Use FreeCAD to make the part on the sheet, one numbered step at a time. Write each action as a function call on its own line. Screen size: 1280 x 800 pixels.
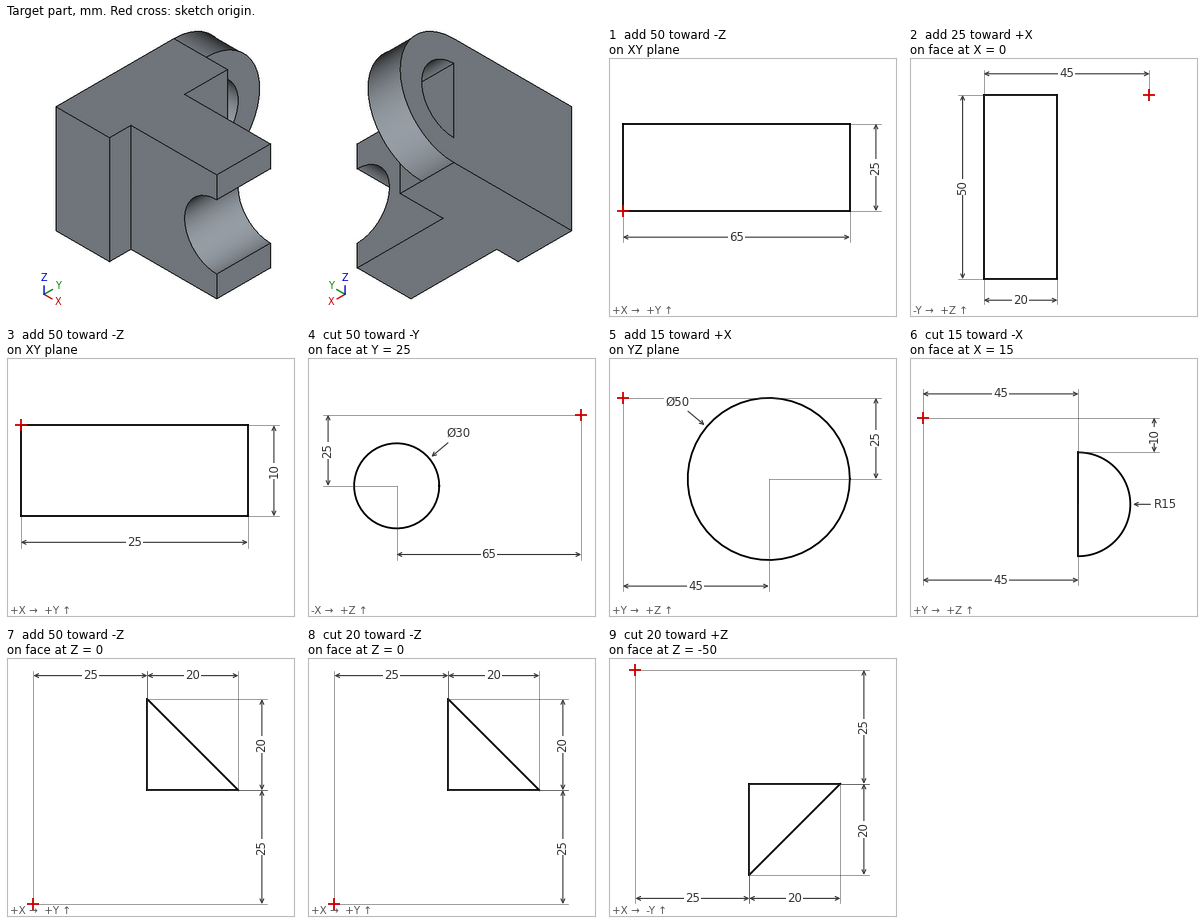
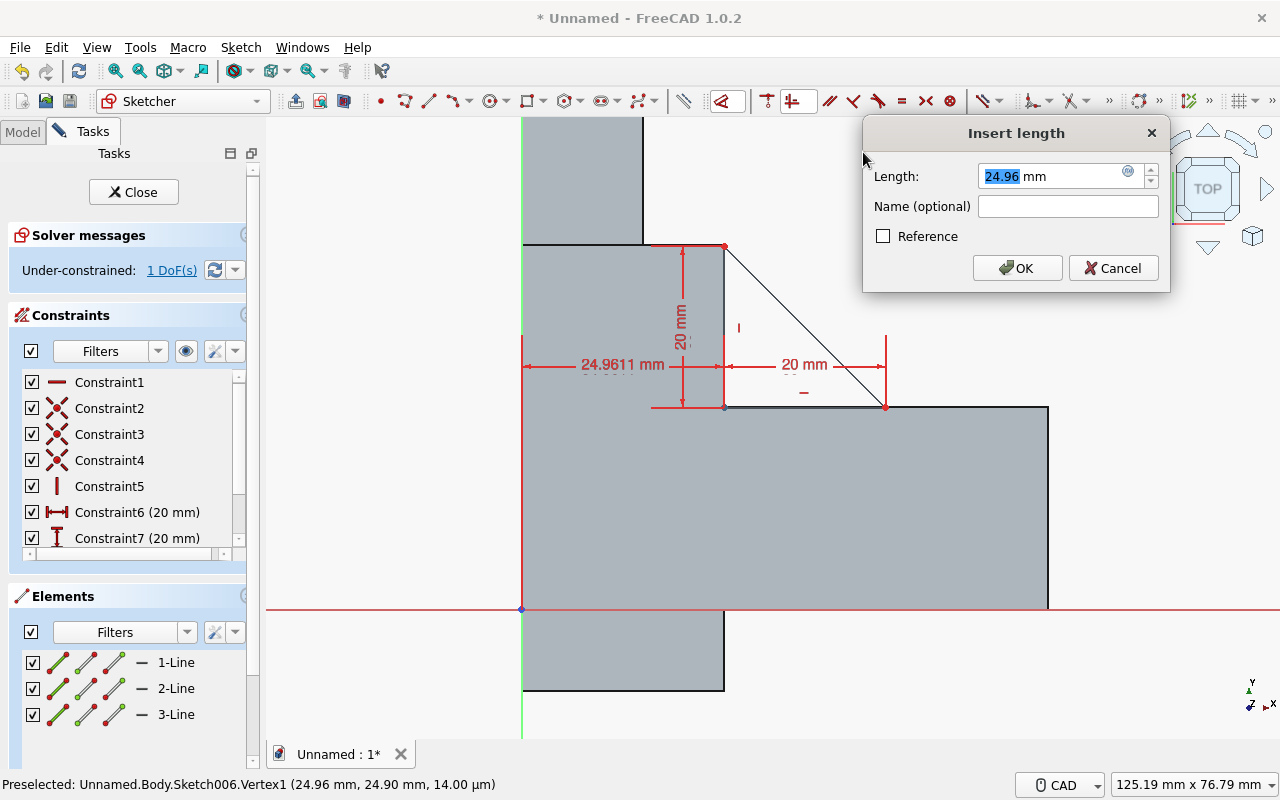
text(25)
key(Return)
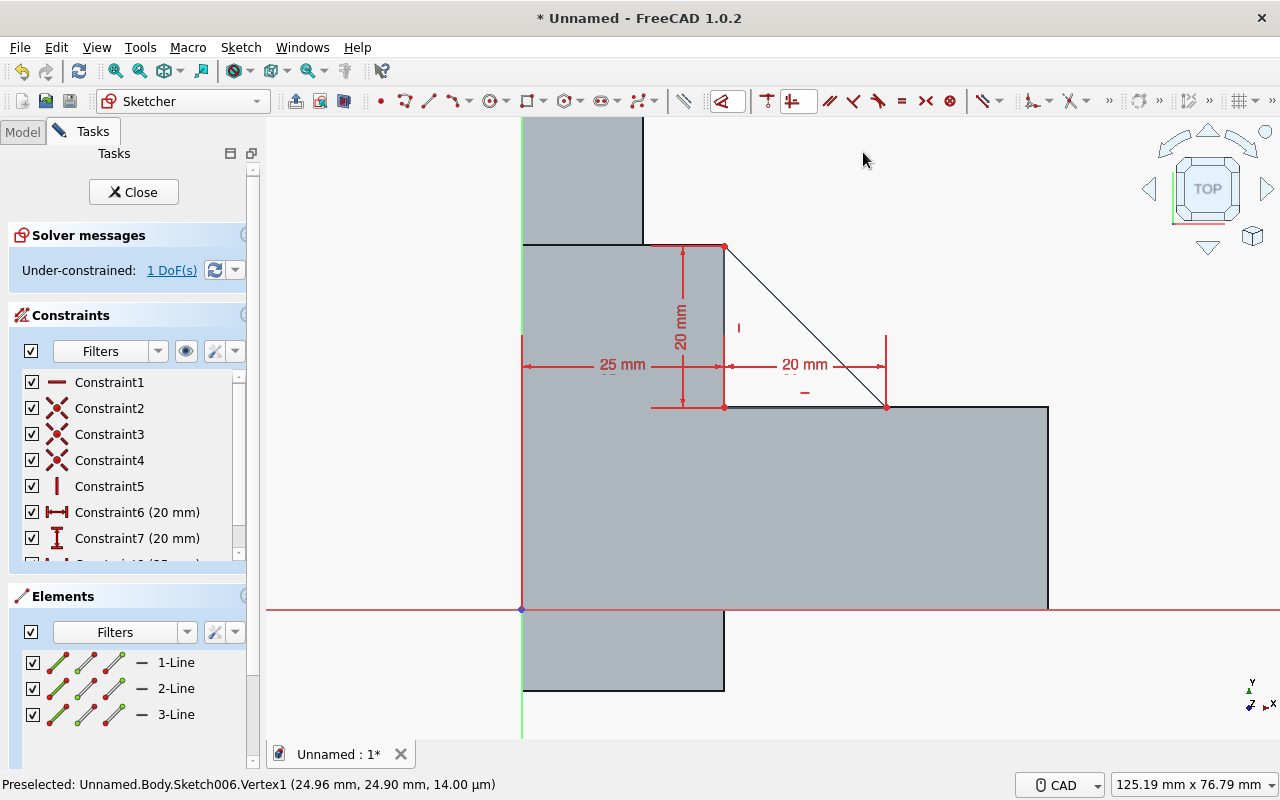
click(724, 408)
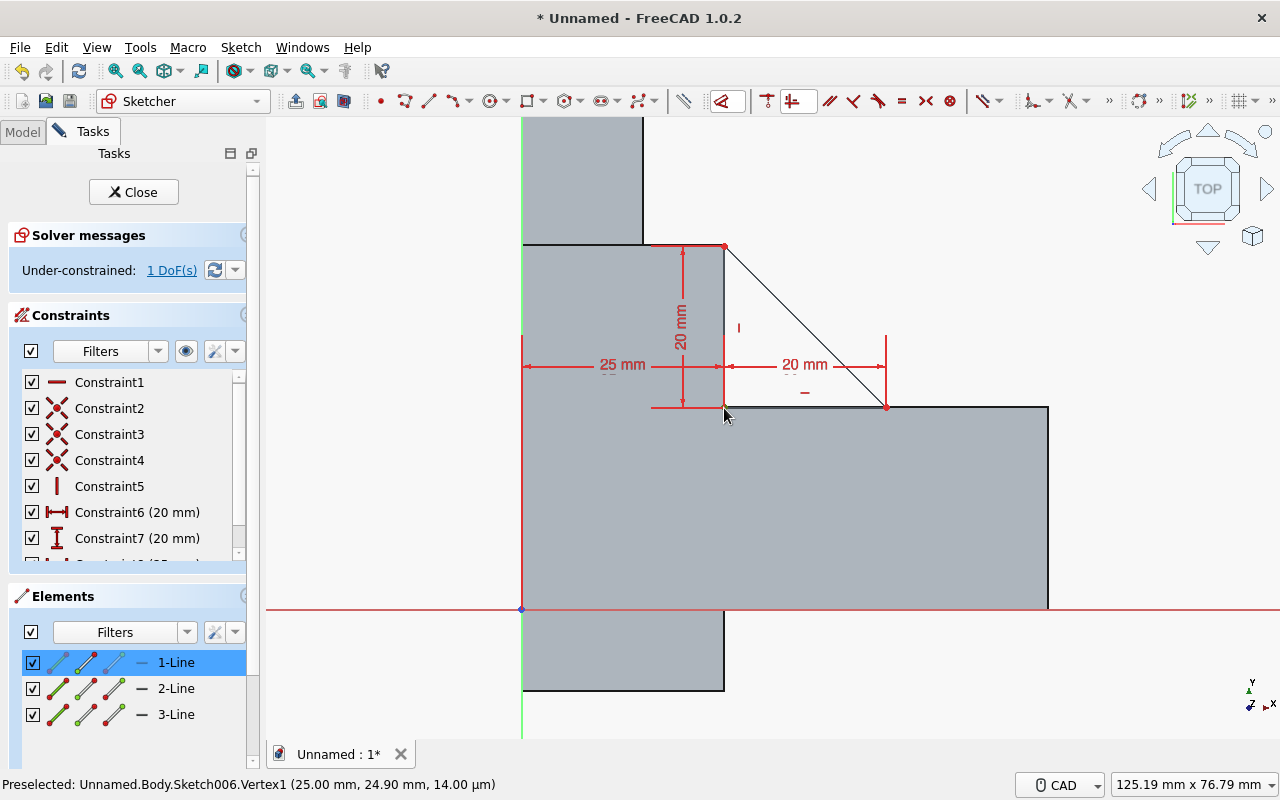
click(740, 102)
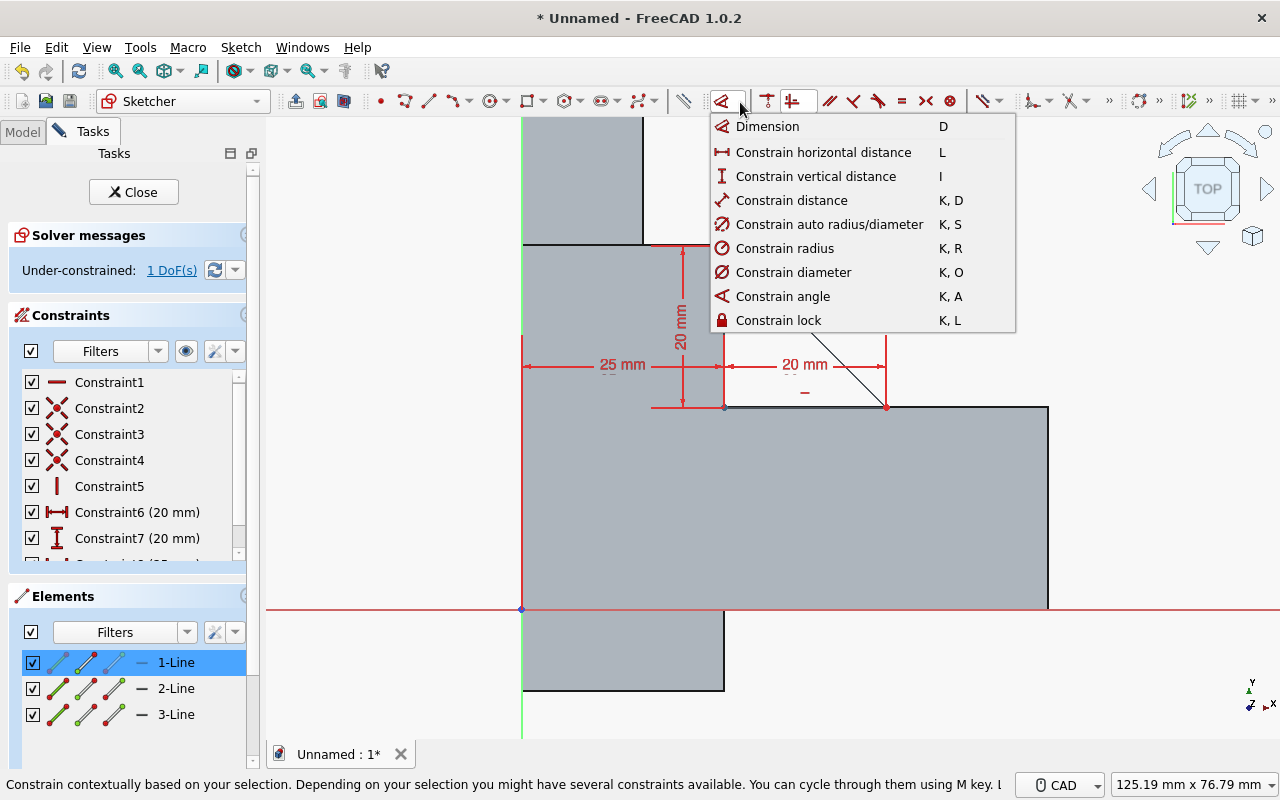
click(863, 176)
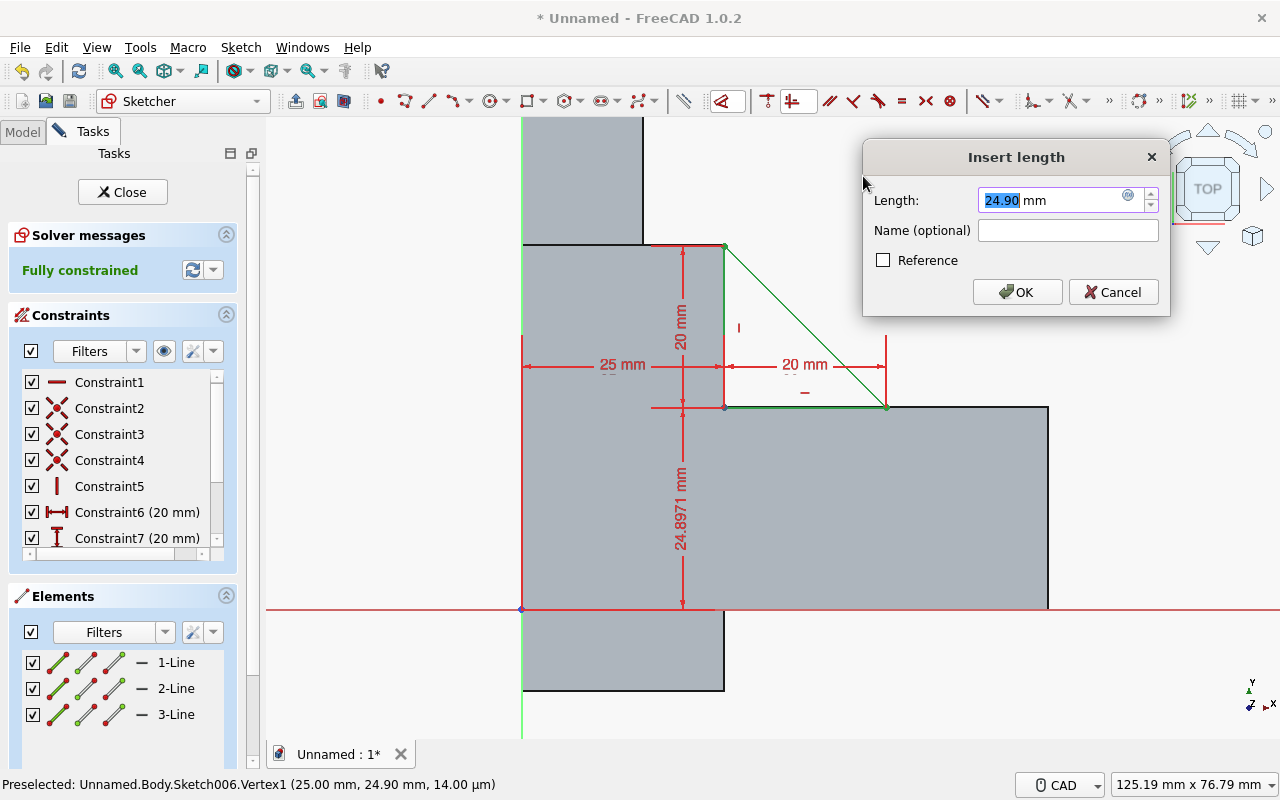
text(25)
key(Return)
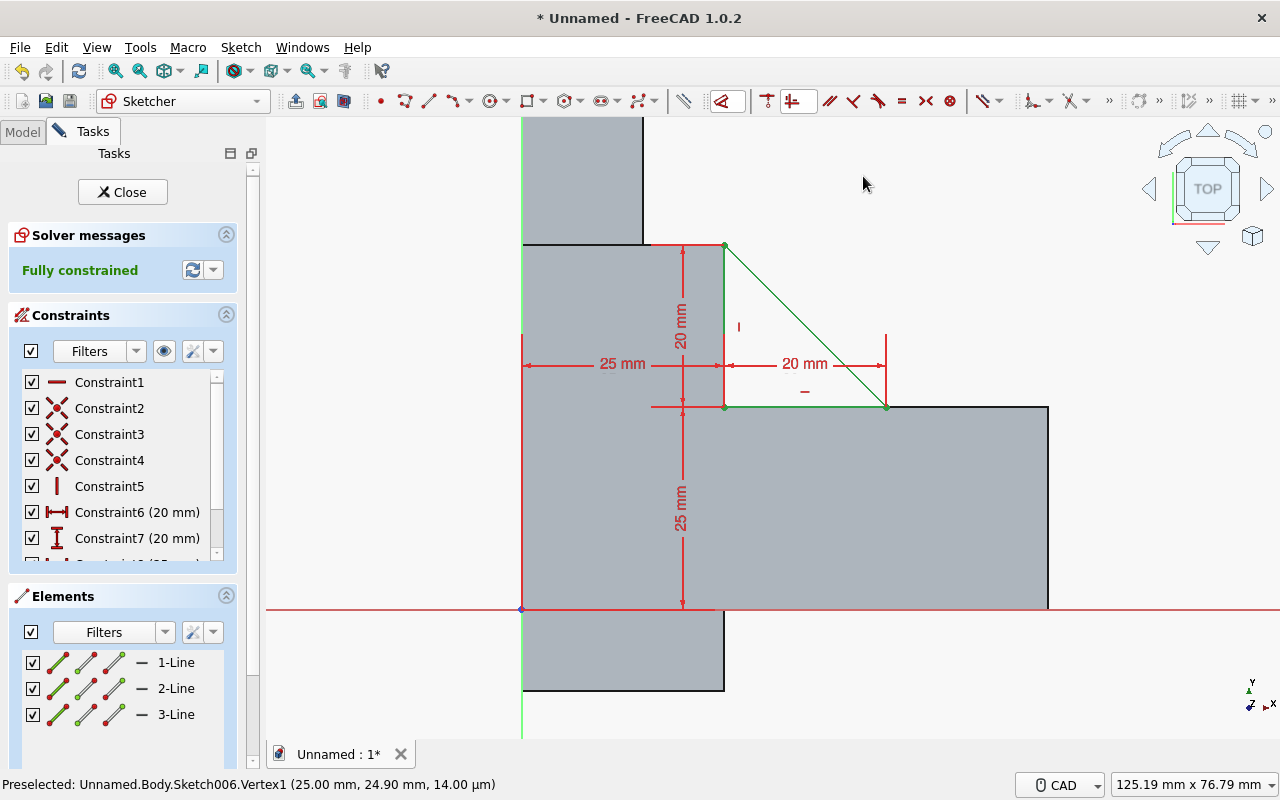
click(123, 192)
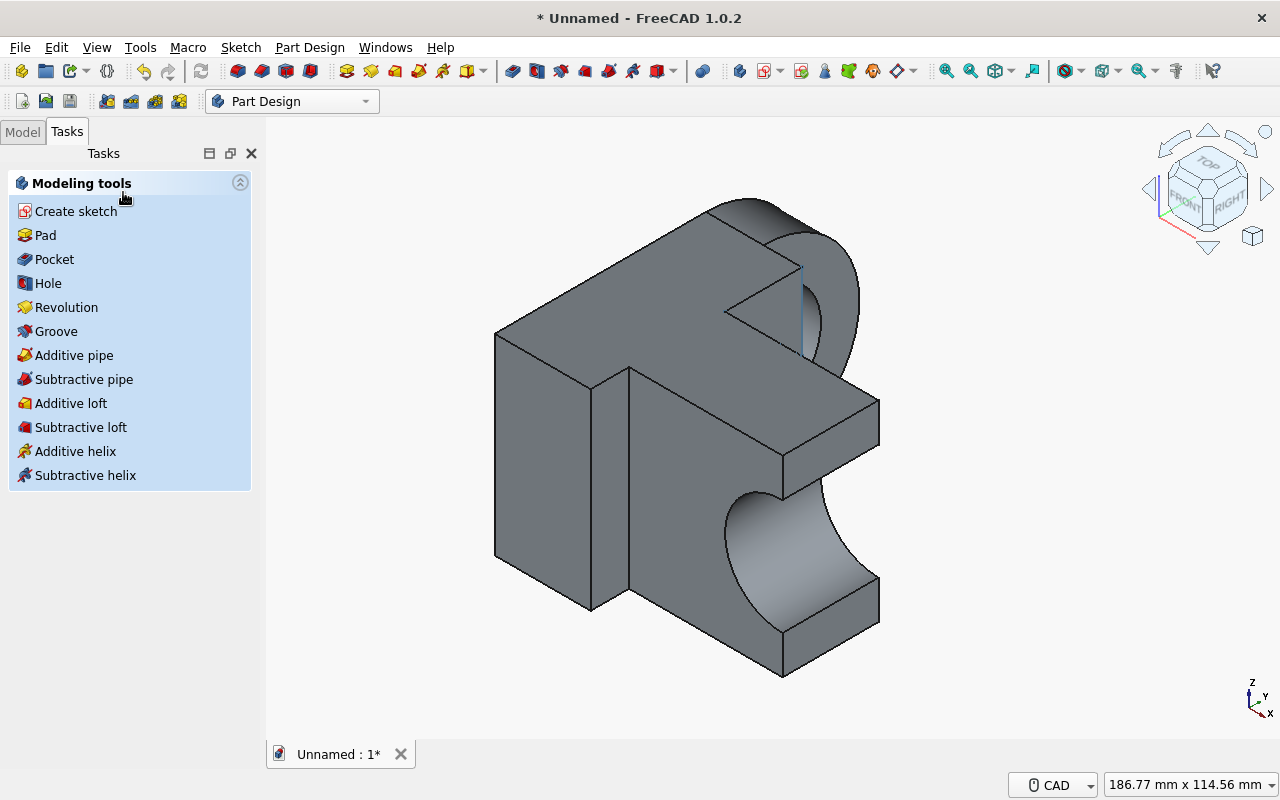
click(348, 72)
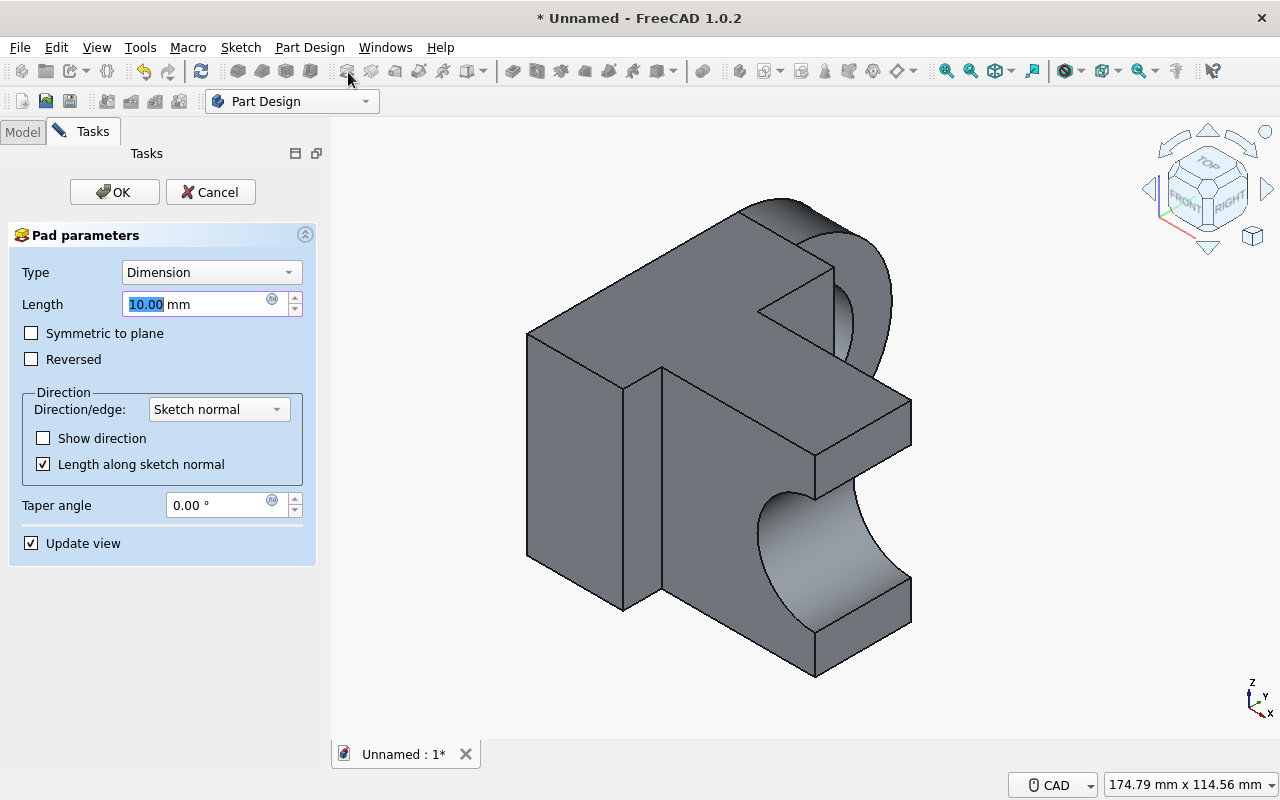
text(50)
key(Tab)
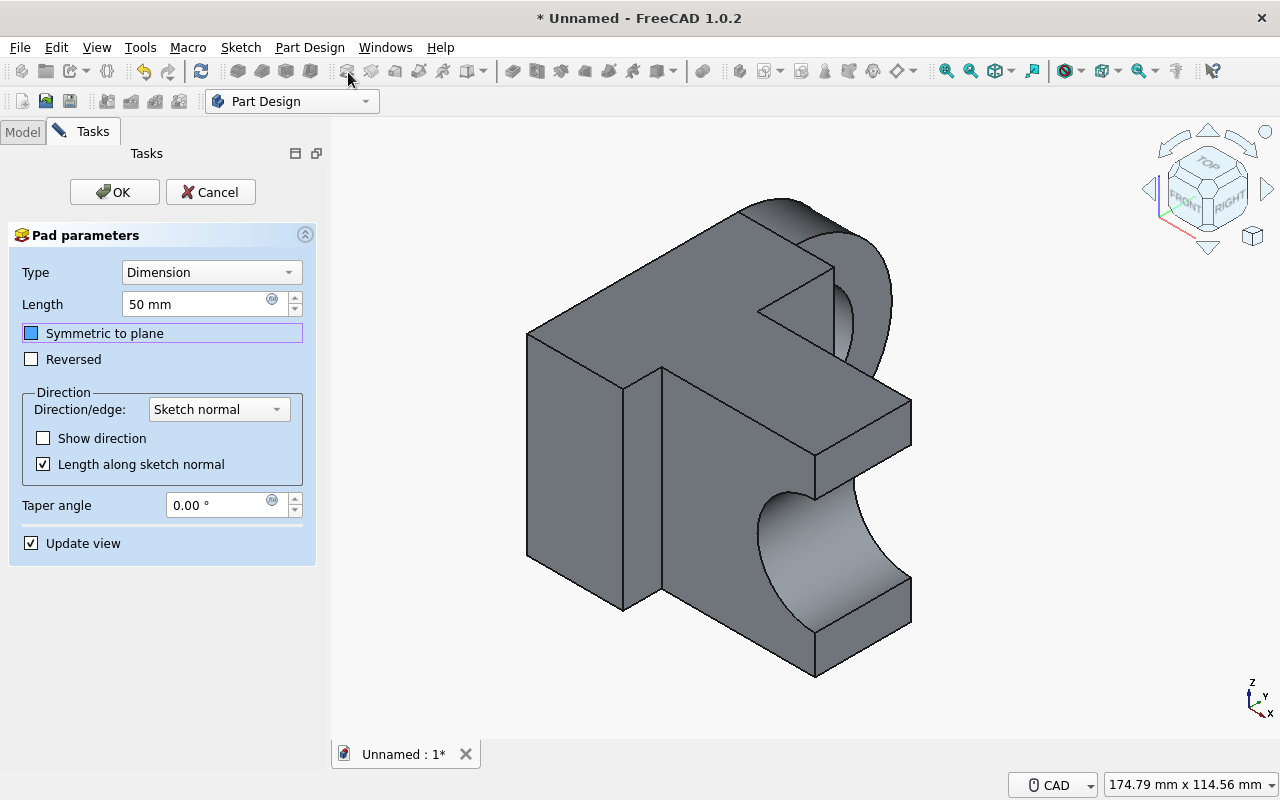
click(30, 359)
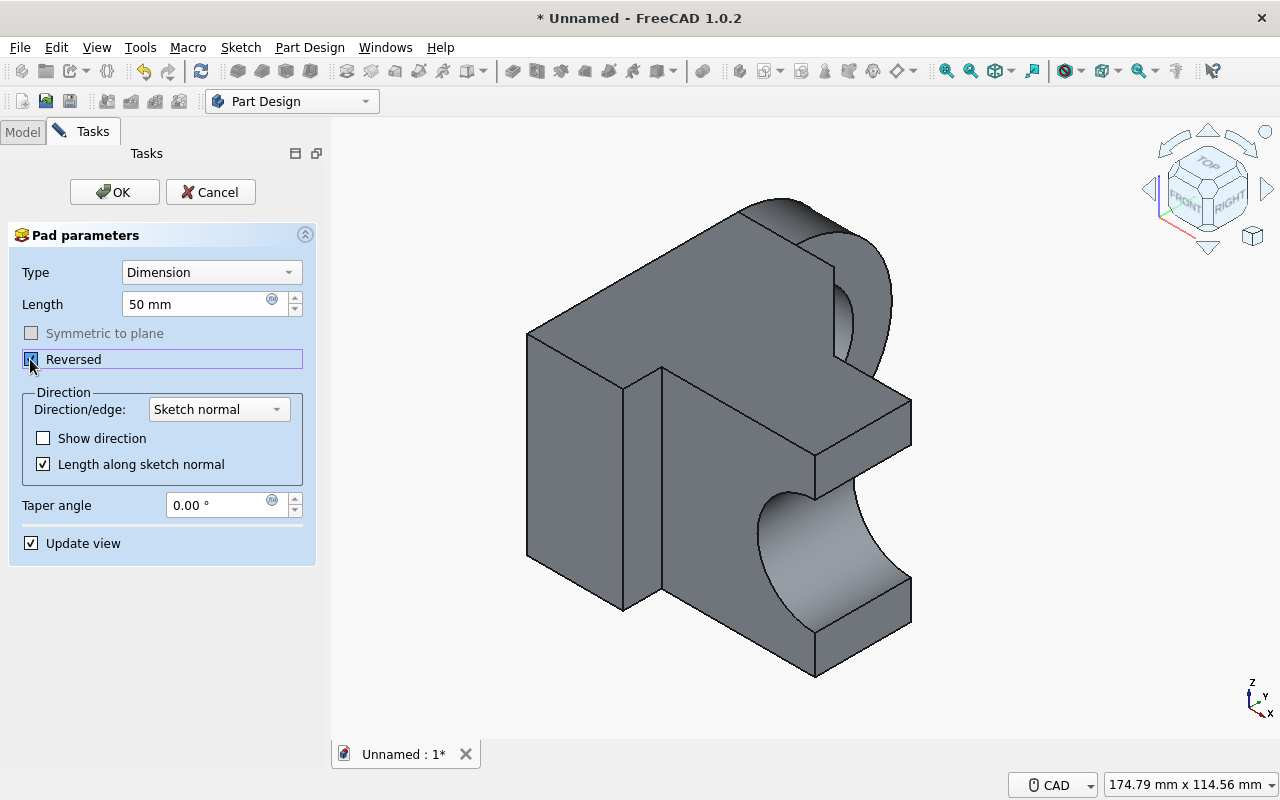
click(115, 192)